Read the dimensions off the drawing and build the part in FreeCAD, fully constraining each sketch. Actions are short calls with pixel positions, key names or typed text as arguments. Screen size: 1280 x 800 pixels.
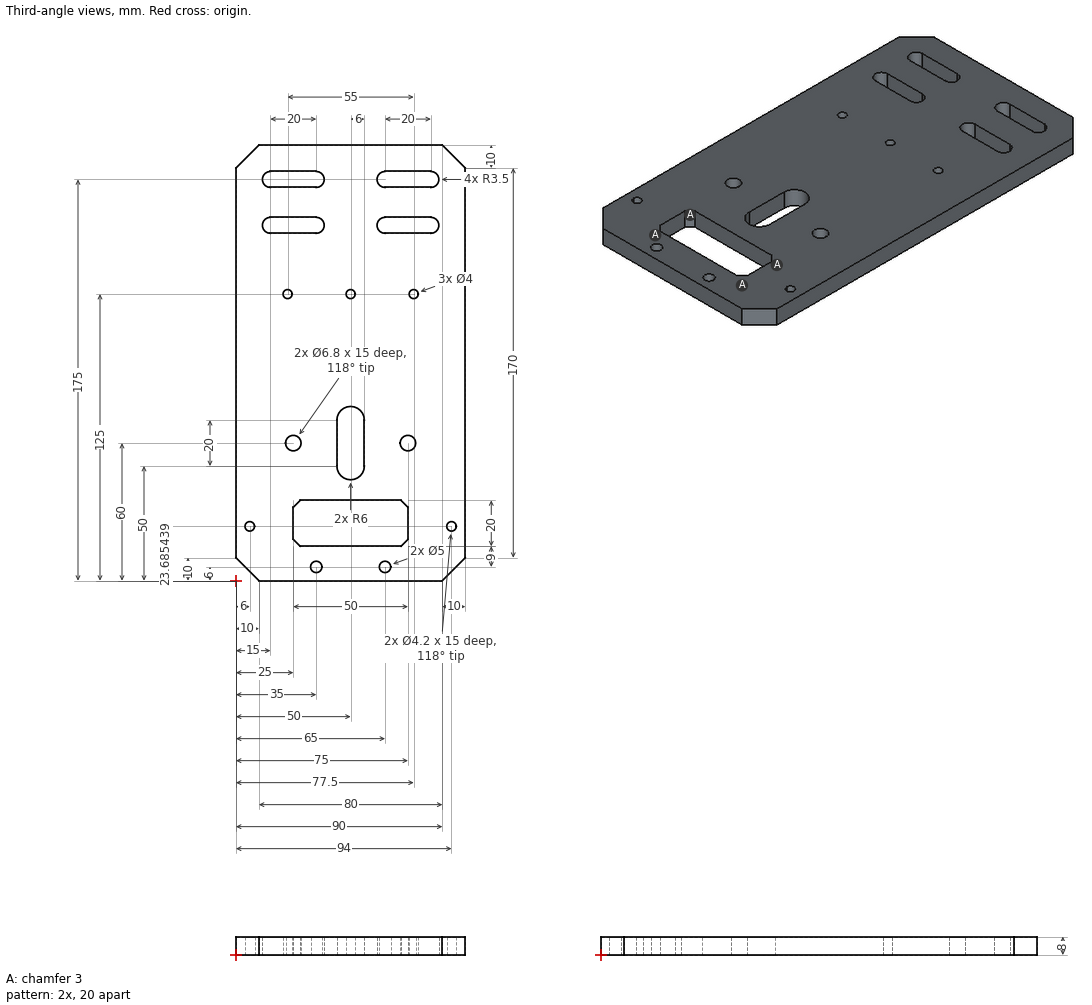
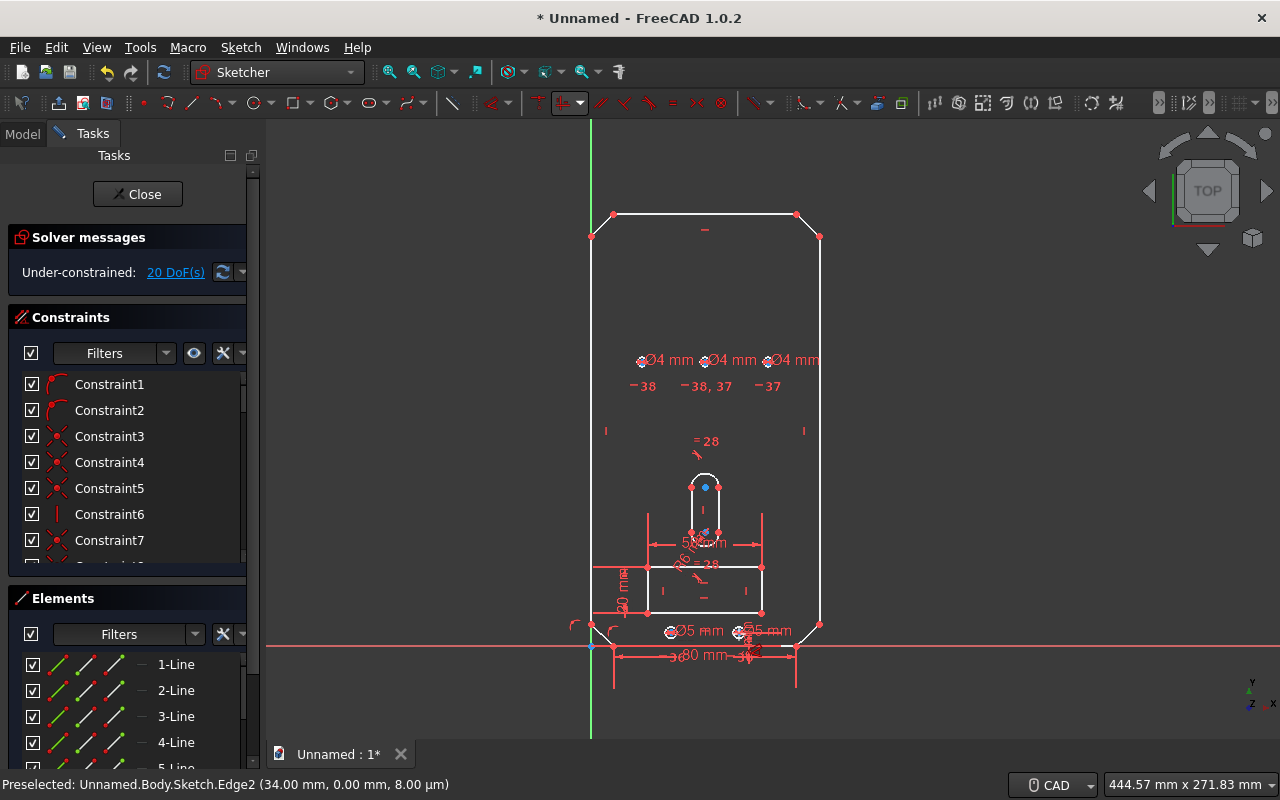
click(742, 214)
click(705, 180)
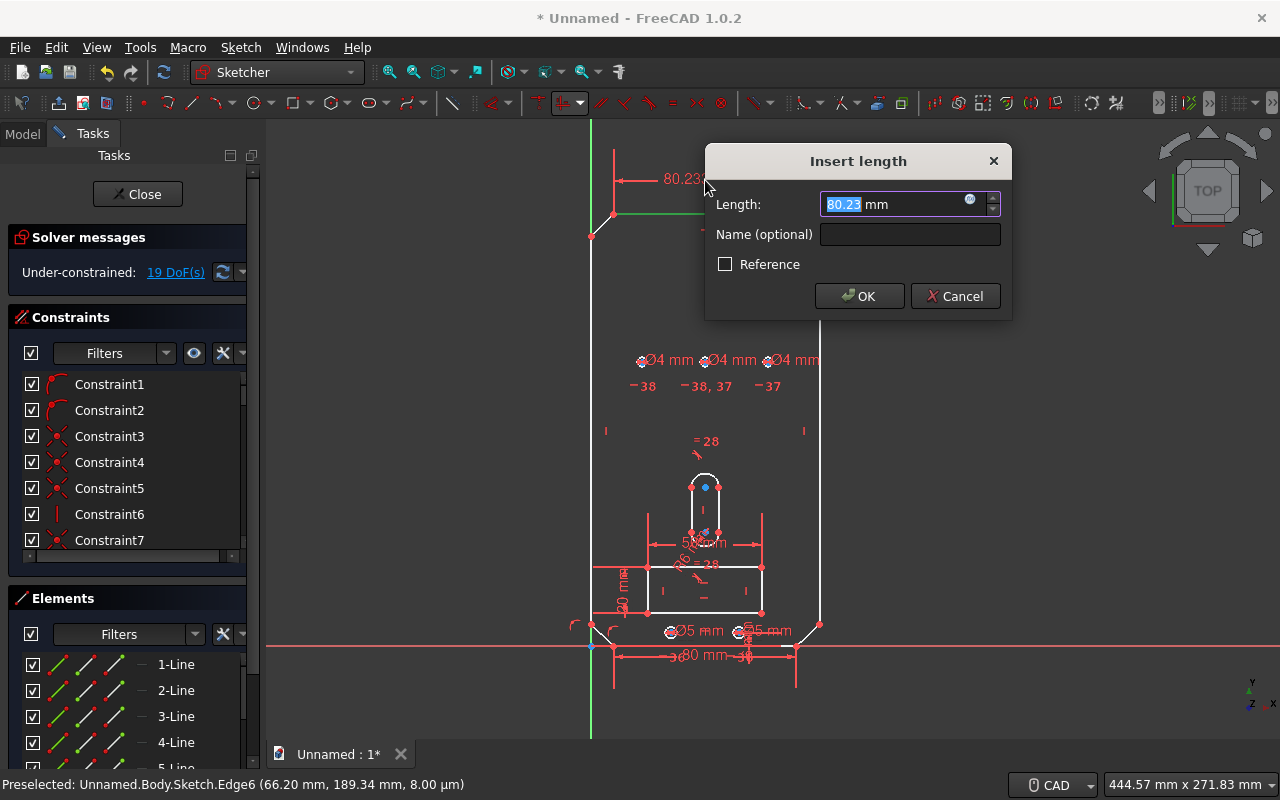
text(80)
key(Return)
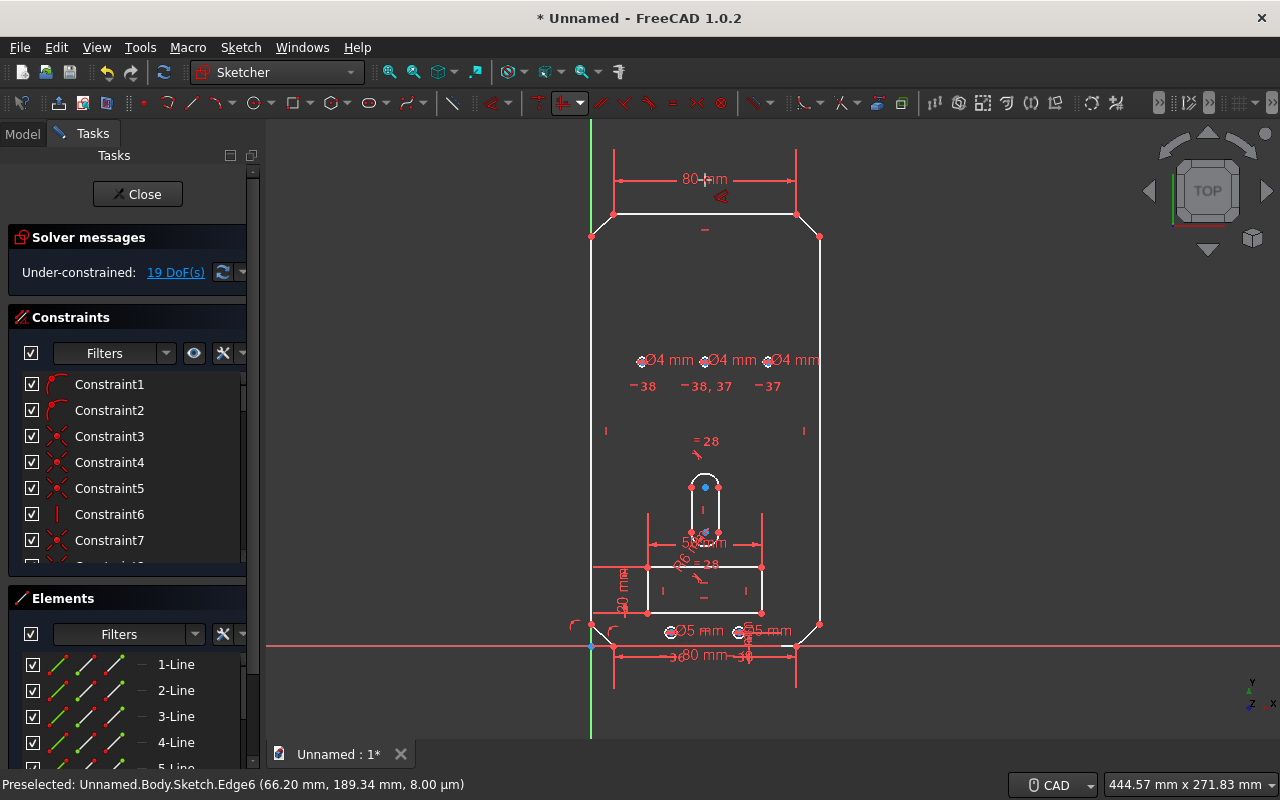
click(692, 519)
click(658, 510)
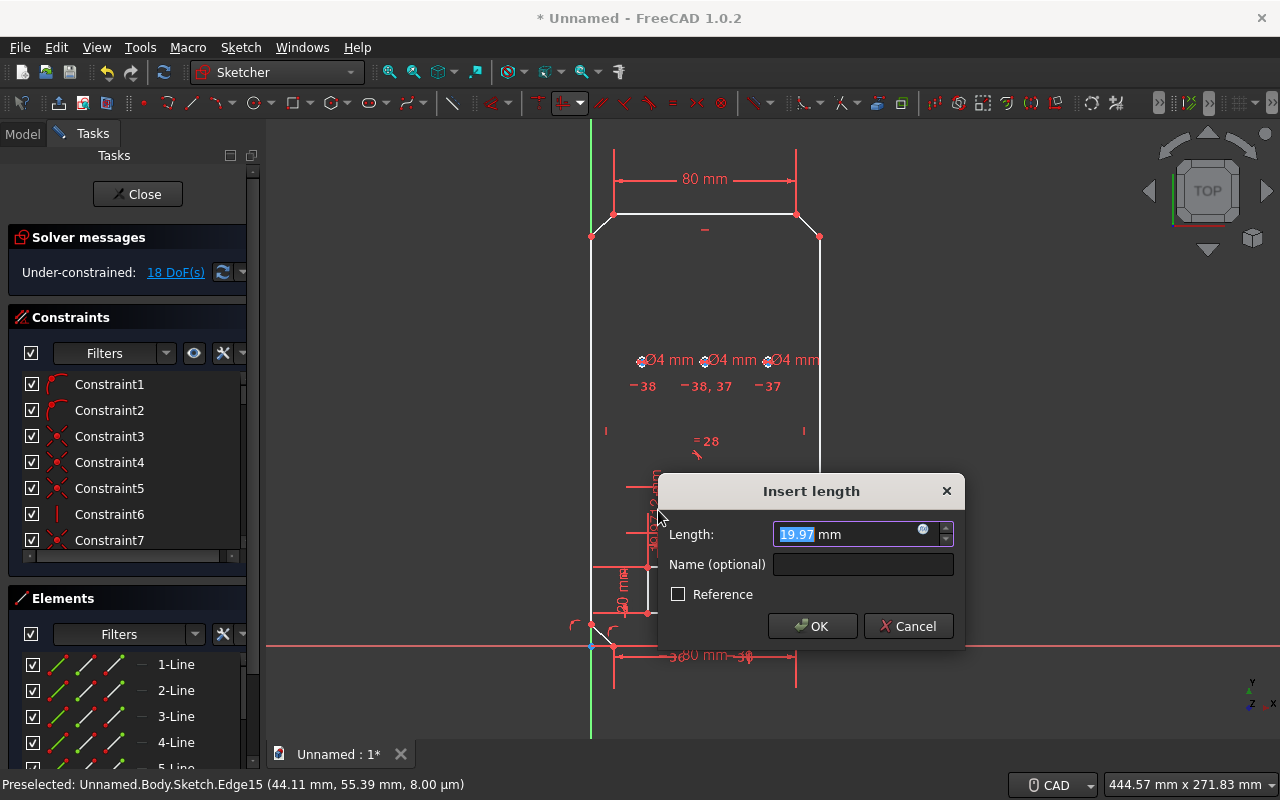
text(20)
key(Return)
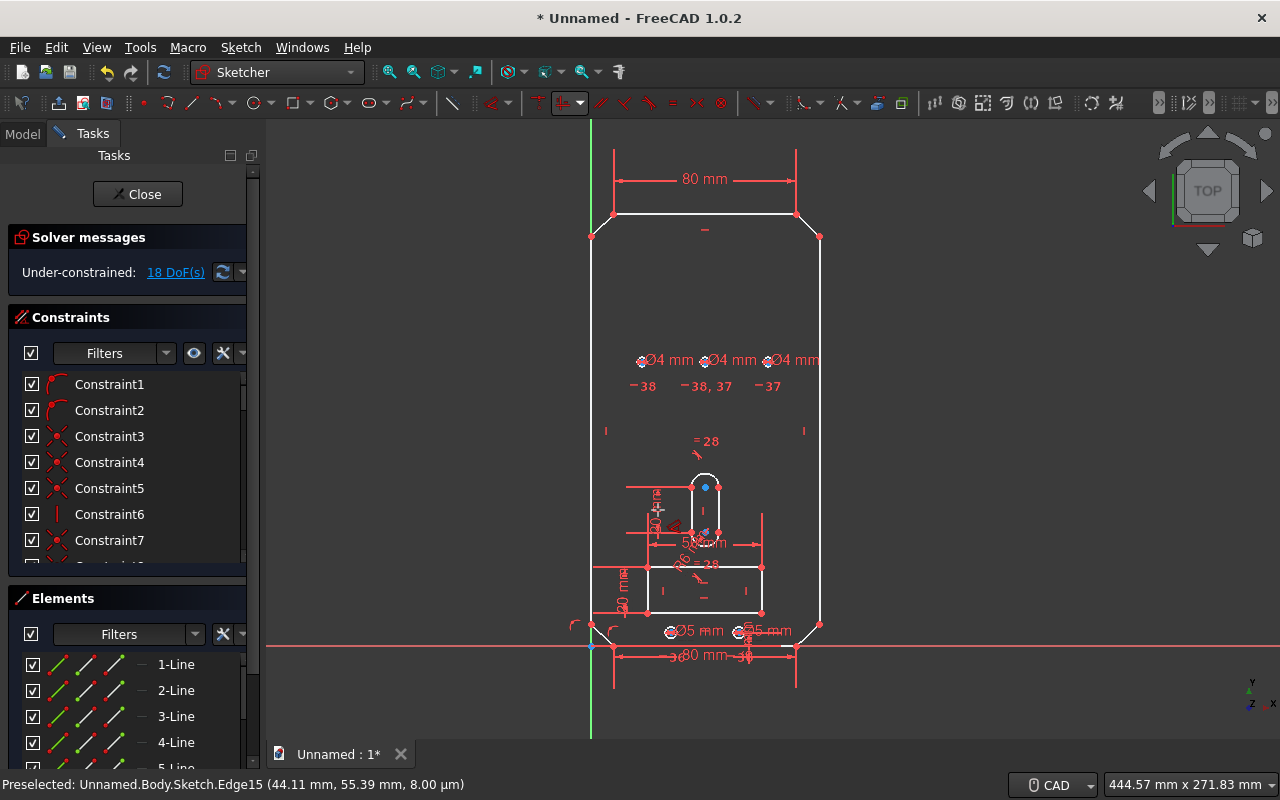
click(739, 633)
click(665, 680)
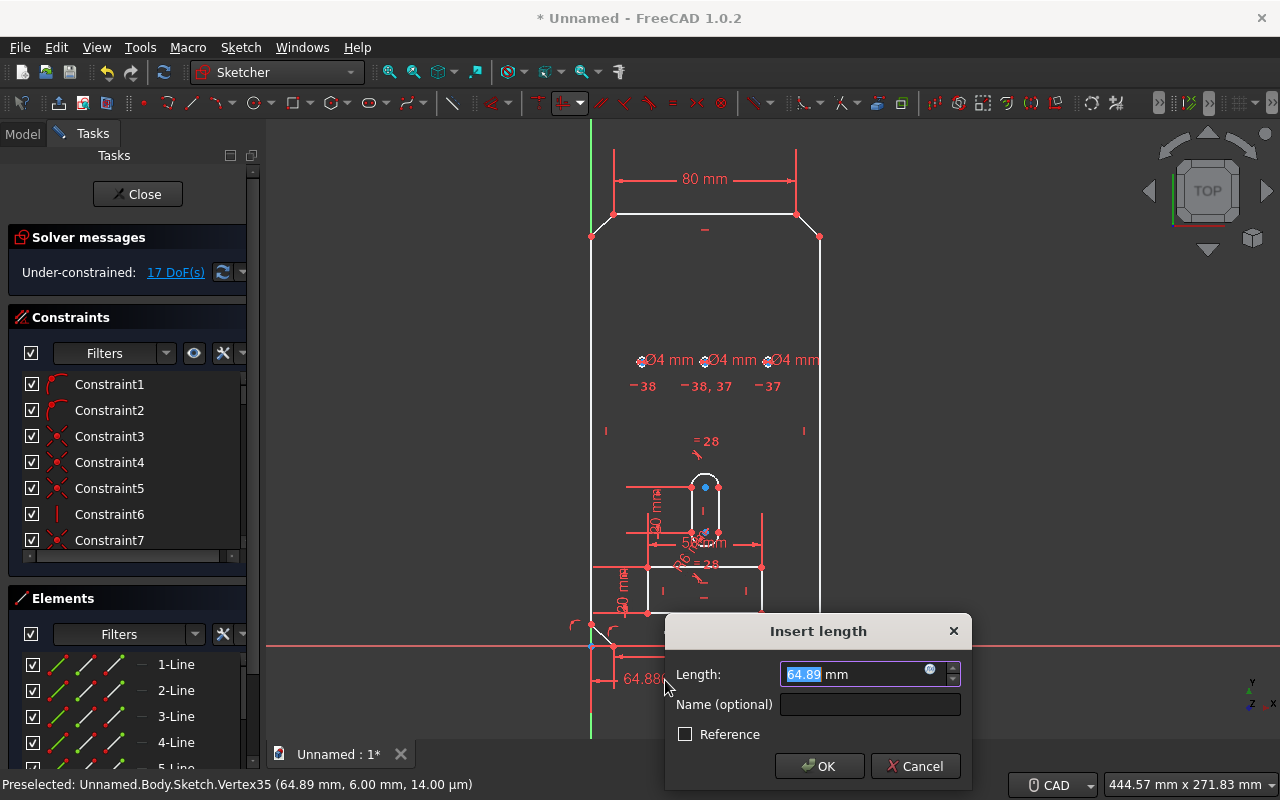
text(65)
key(Return)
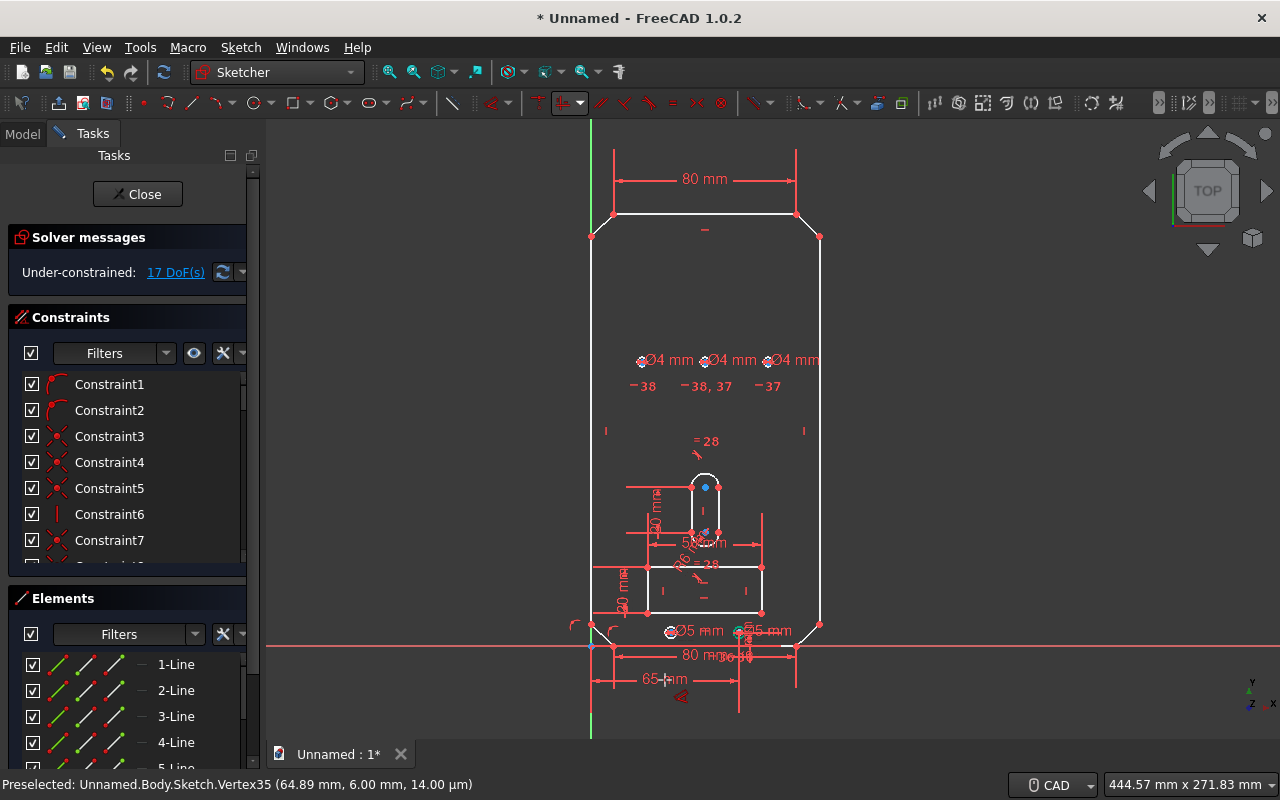
click(671, 633)
click(631, 599)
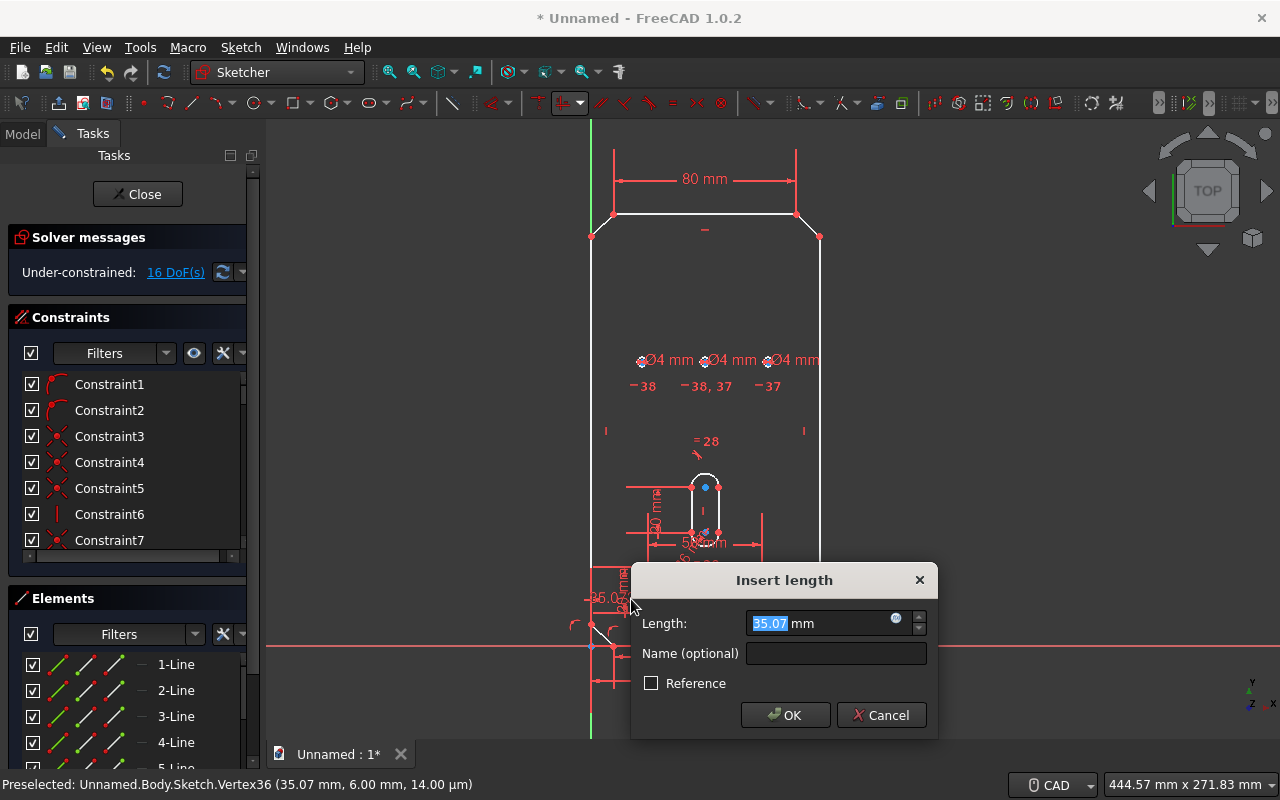
text(35)
key(Return)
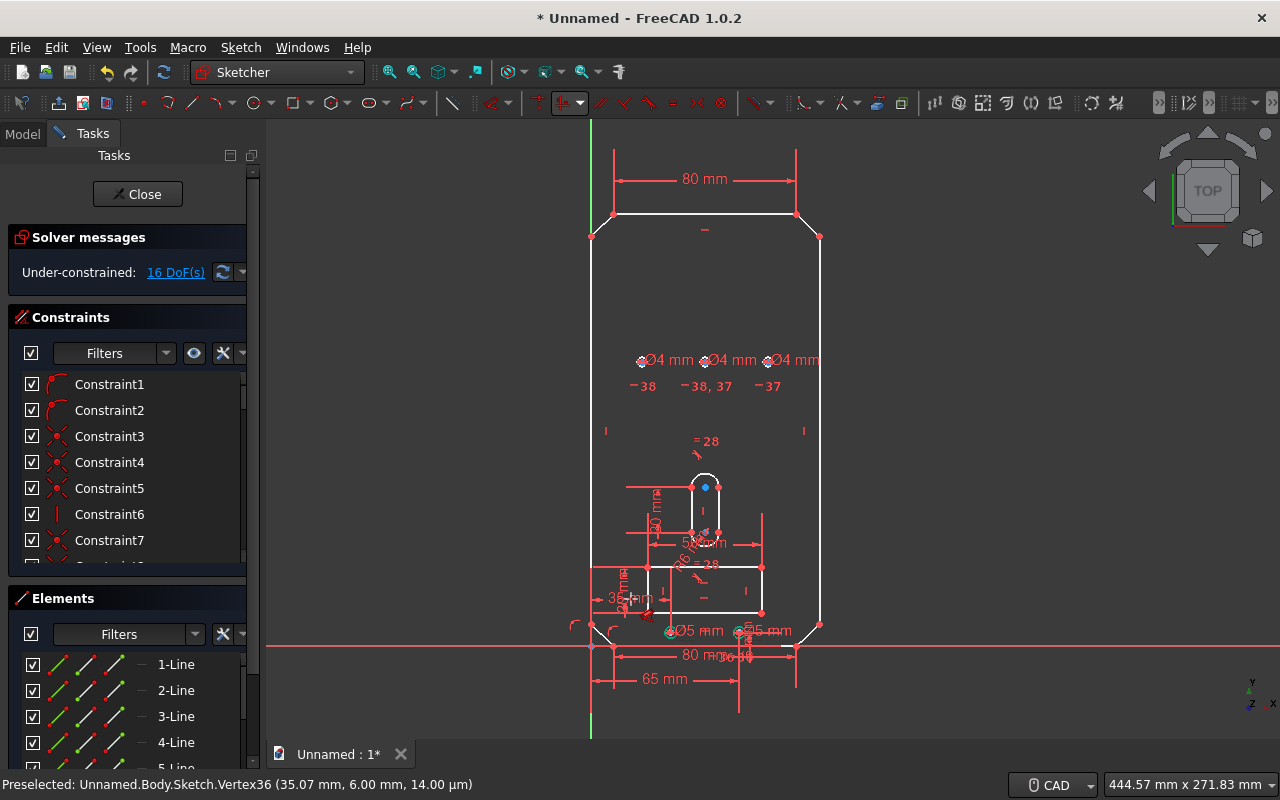
click(705, 362)
click(648, 328)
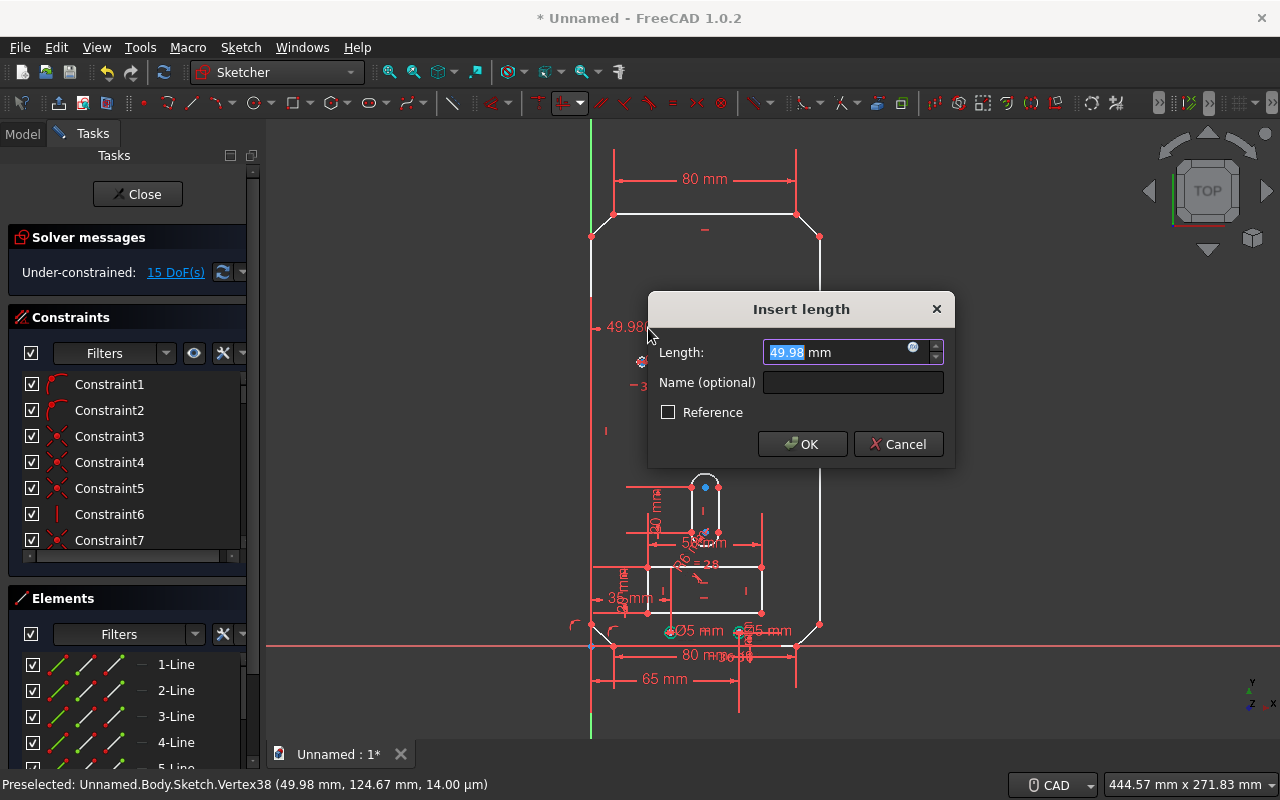
text(50)
key(Return)